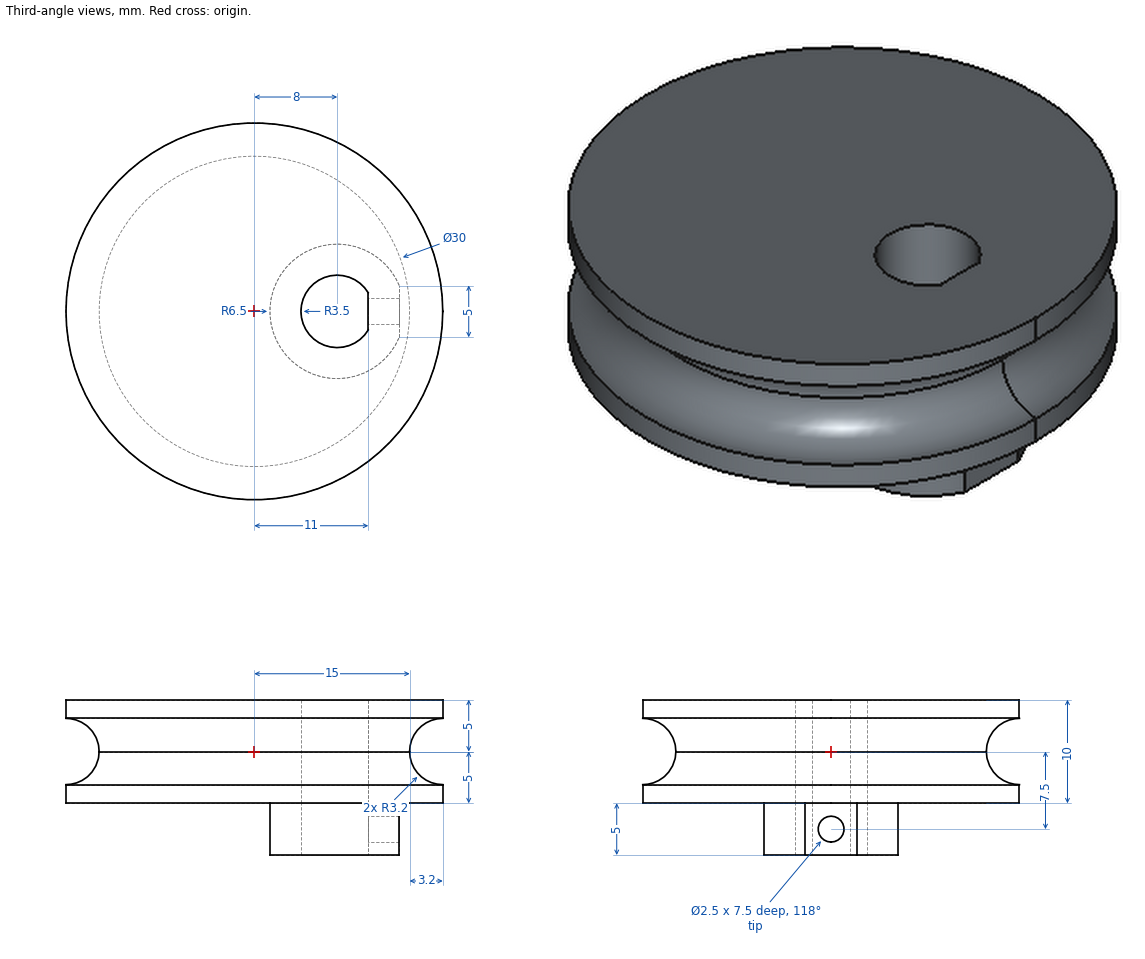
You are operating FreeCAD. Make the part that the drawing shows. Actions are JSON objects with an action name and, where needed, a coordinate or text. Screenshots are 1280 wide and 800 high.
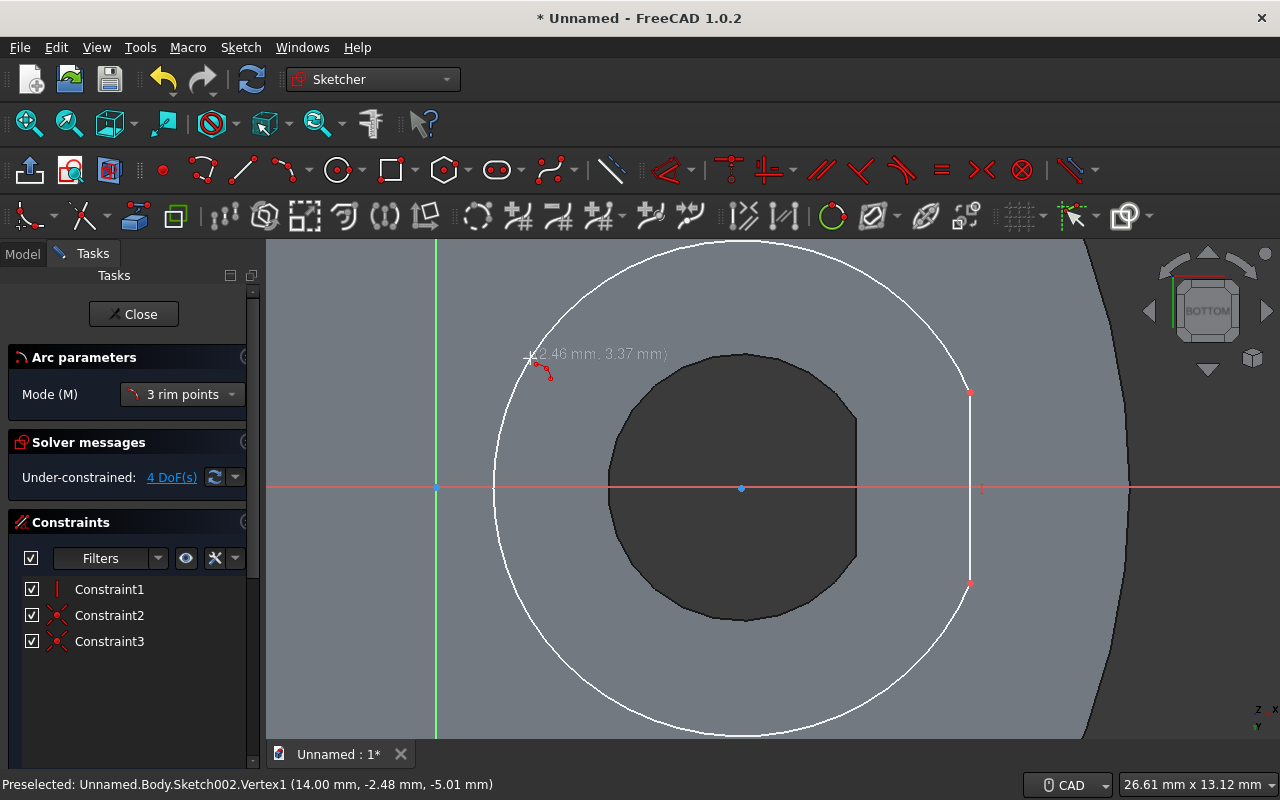
{"action": "left_click", "coordinate": [244, 170]}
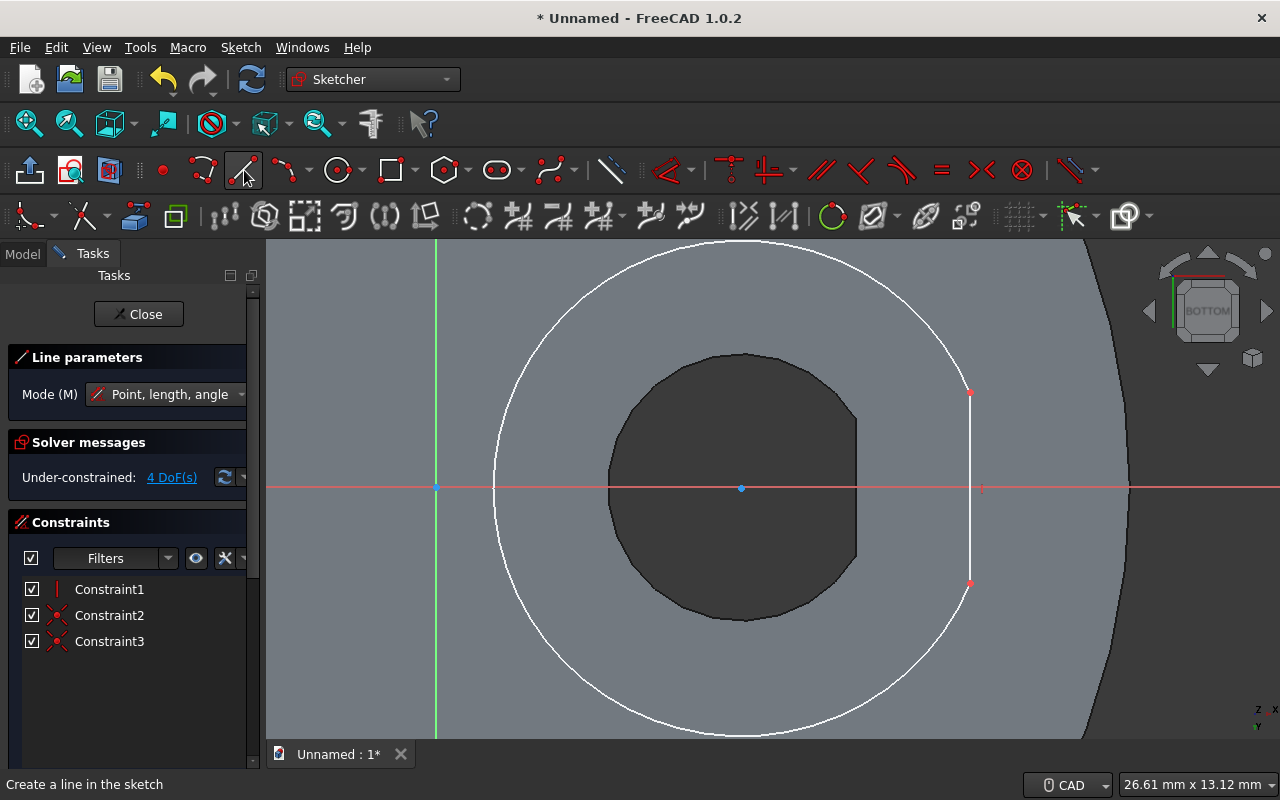
{"action": "left_click", "coordinate": [856, 556]}
{"action": "left_click", "coordinate": [856, 419]}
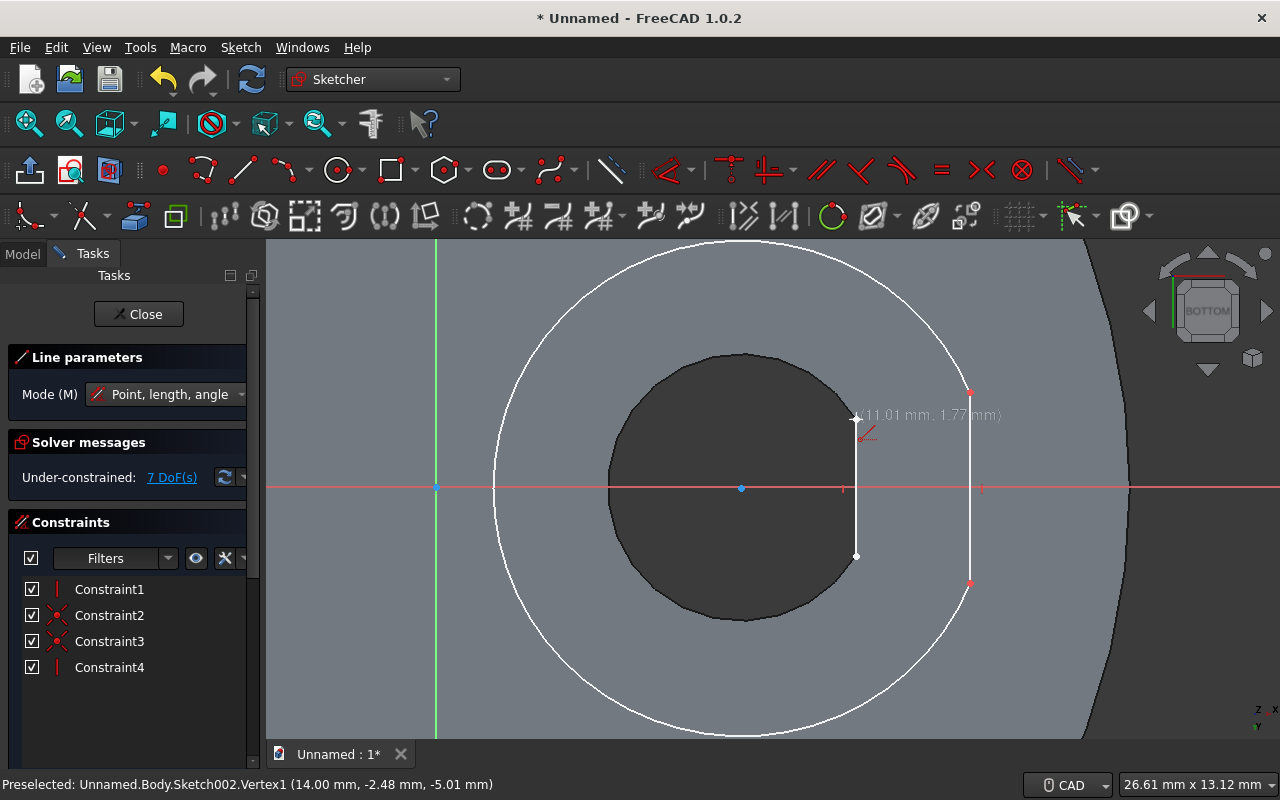
{"action": "left_click", "coordinate": [284, 170]}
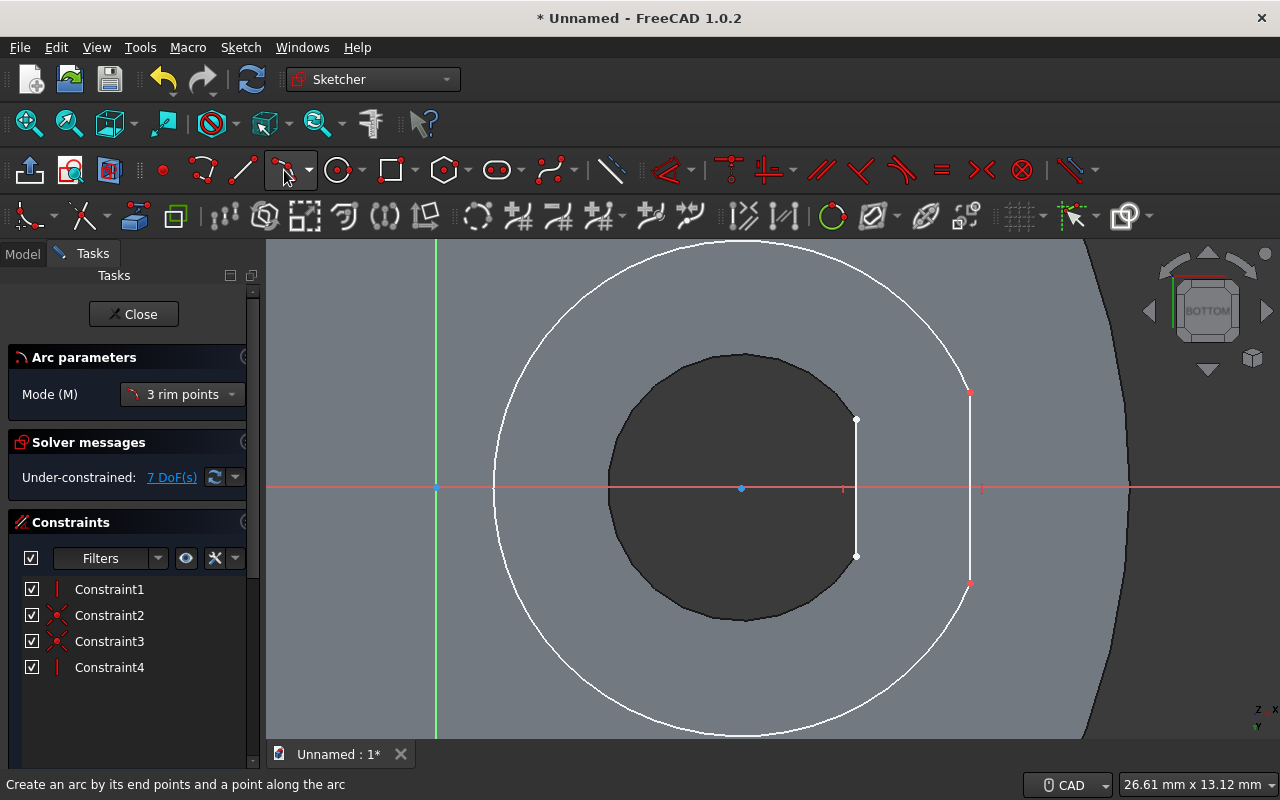
{"action": "left_click", "coordinate": [856, 420]}
{"action": "left_click", "coordinate": [856, 557]}
{"action": "left_click", "coordinate": [626, 421]}
{"action": "key", "text": "Escape"}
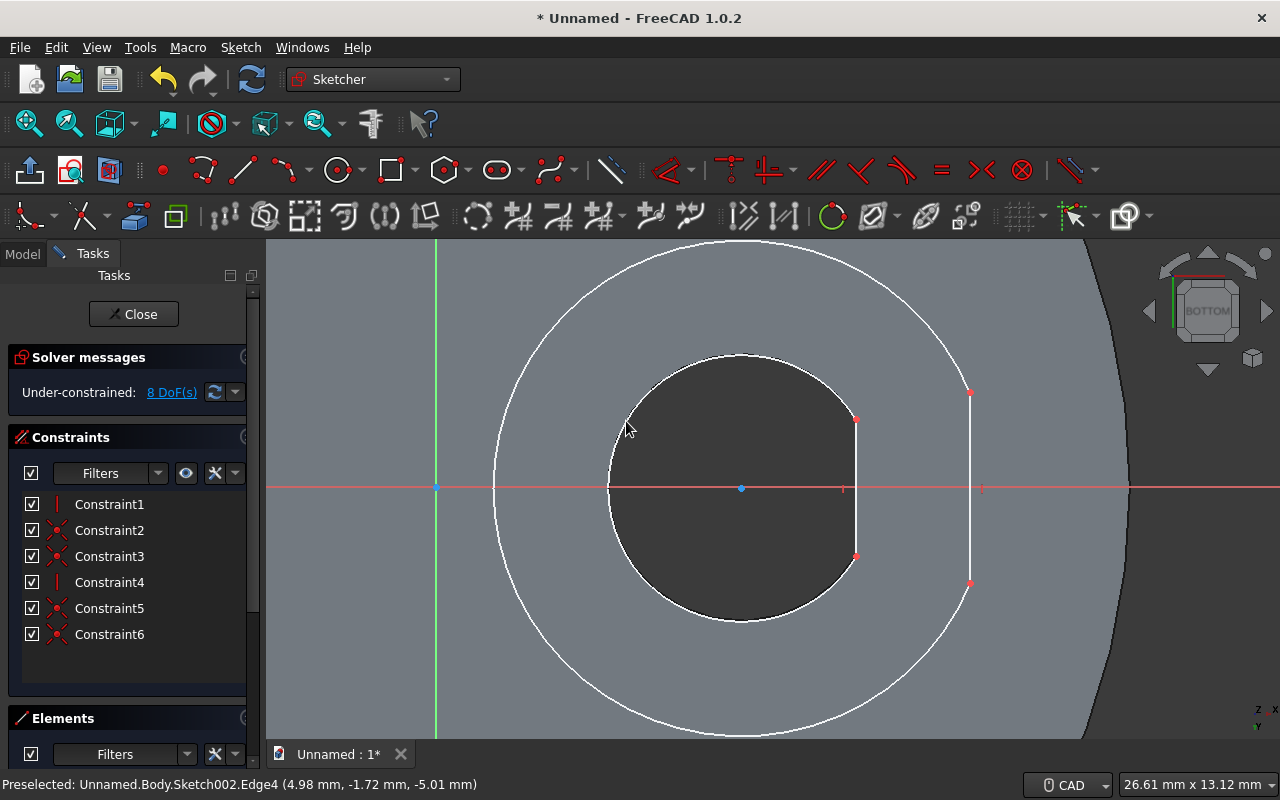
{"action": "left_click", "coordinate": [629, 268]}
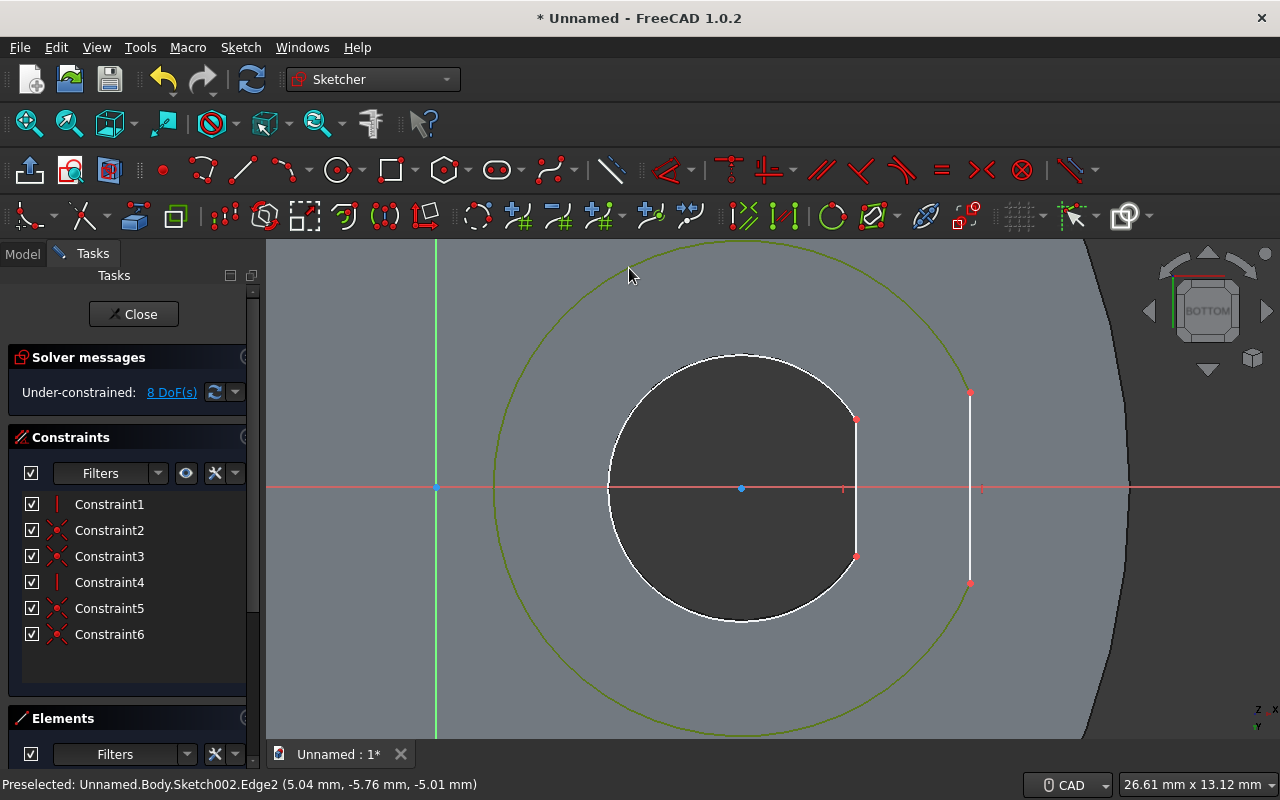
{"action": "left_click", "coordinate": [674, 373]}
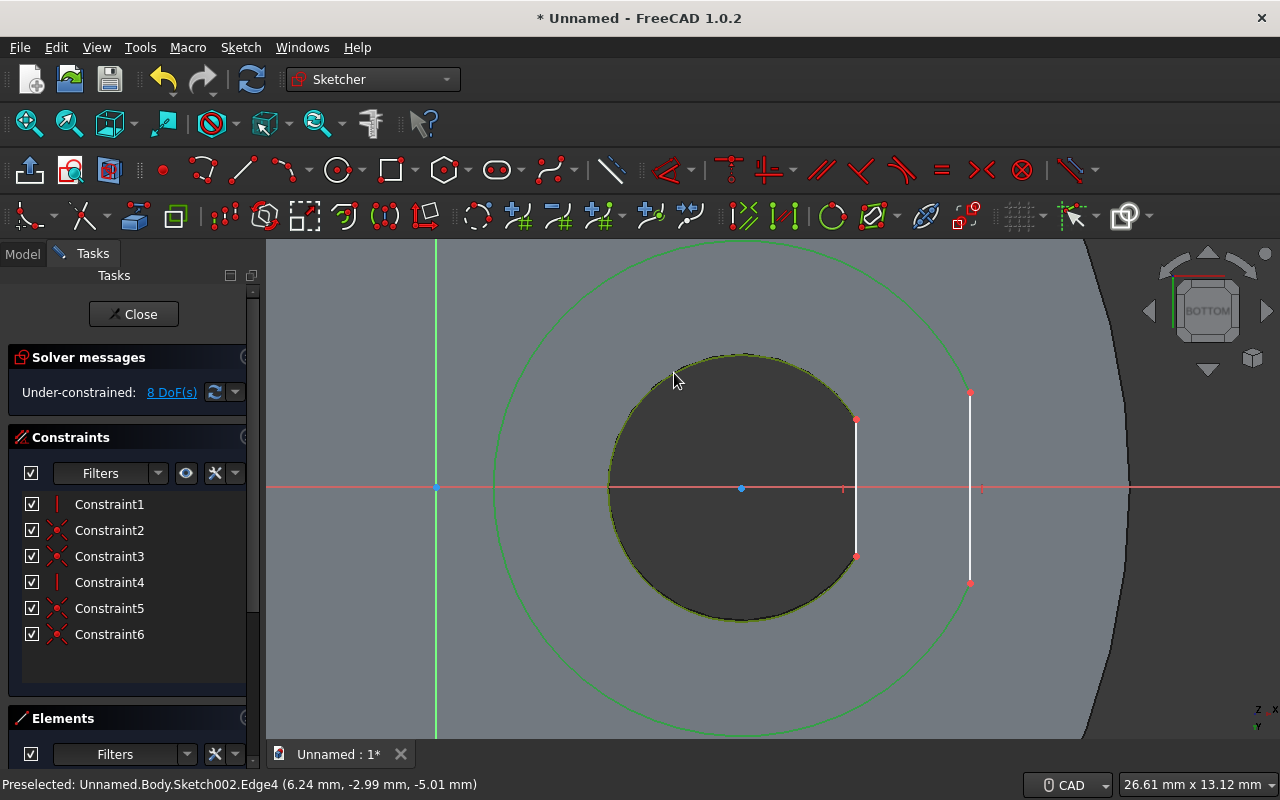
{"action": "left_click", "coordinate": [730, 170]}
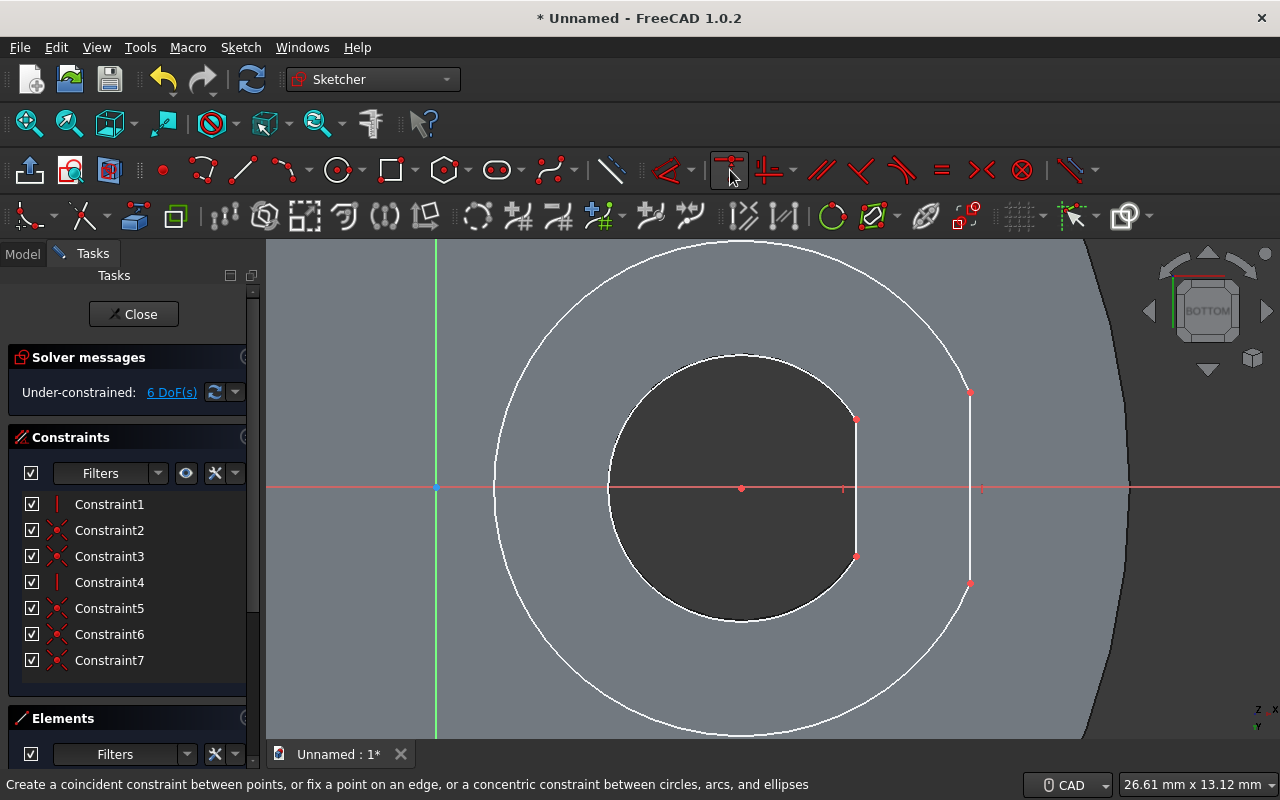
{"action": "left_click", "coordinate": [742, 488]}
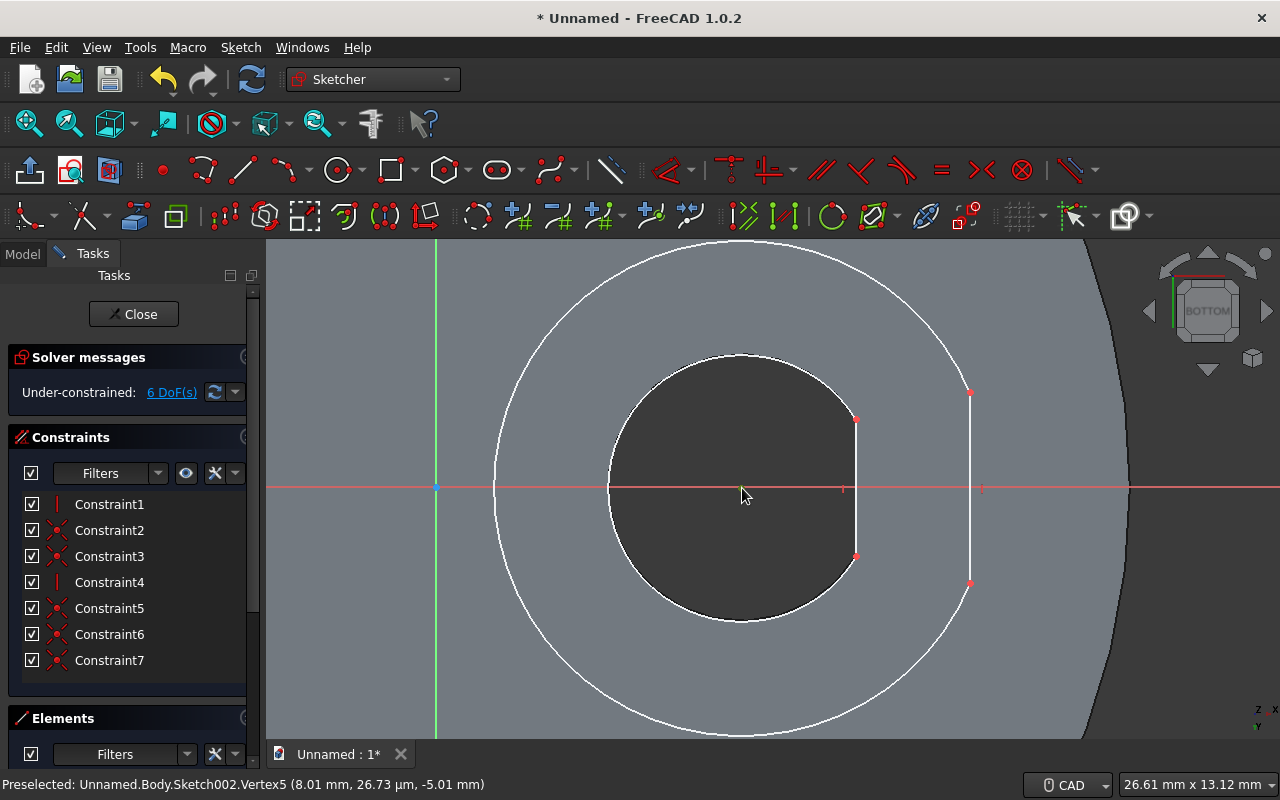
{"action": "left_click", "coordinate": [353, 487]}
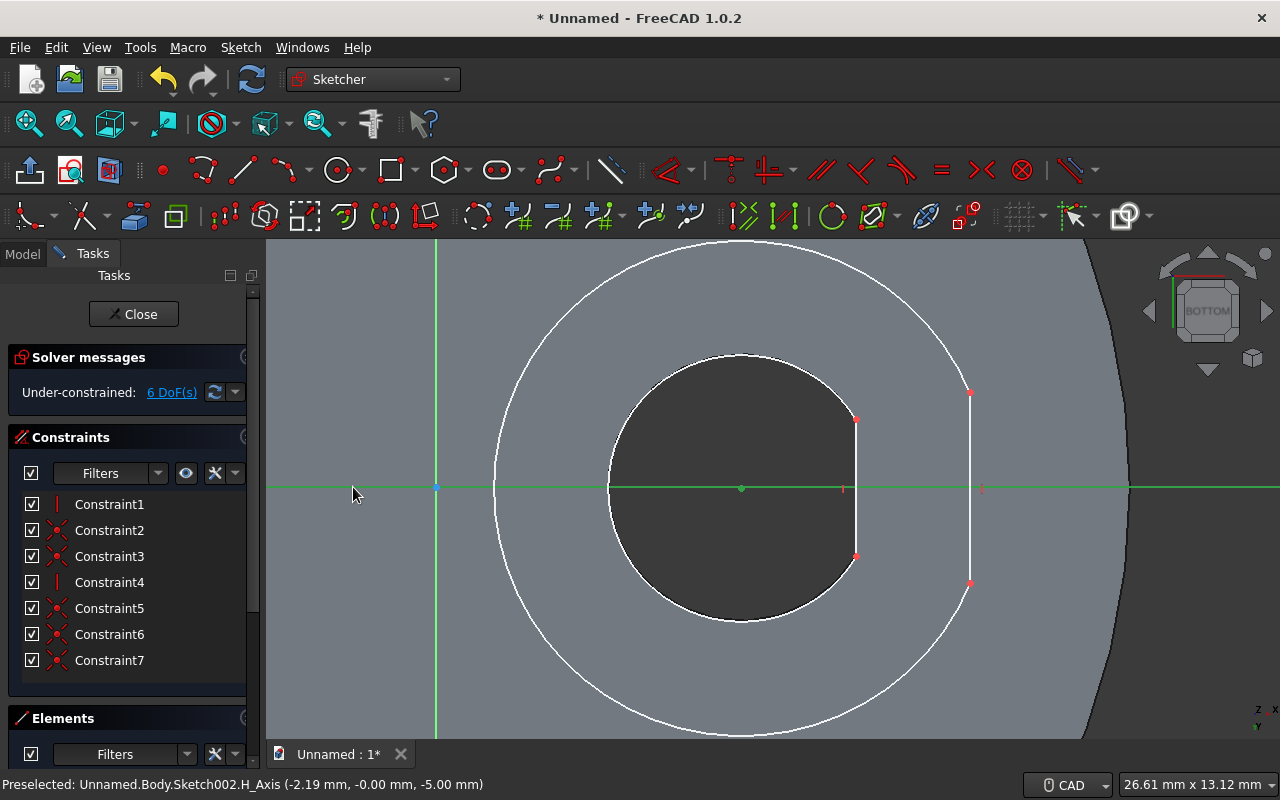
{"action": "left_click", "coordinate": [730, 170]}